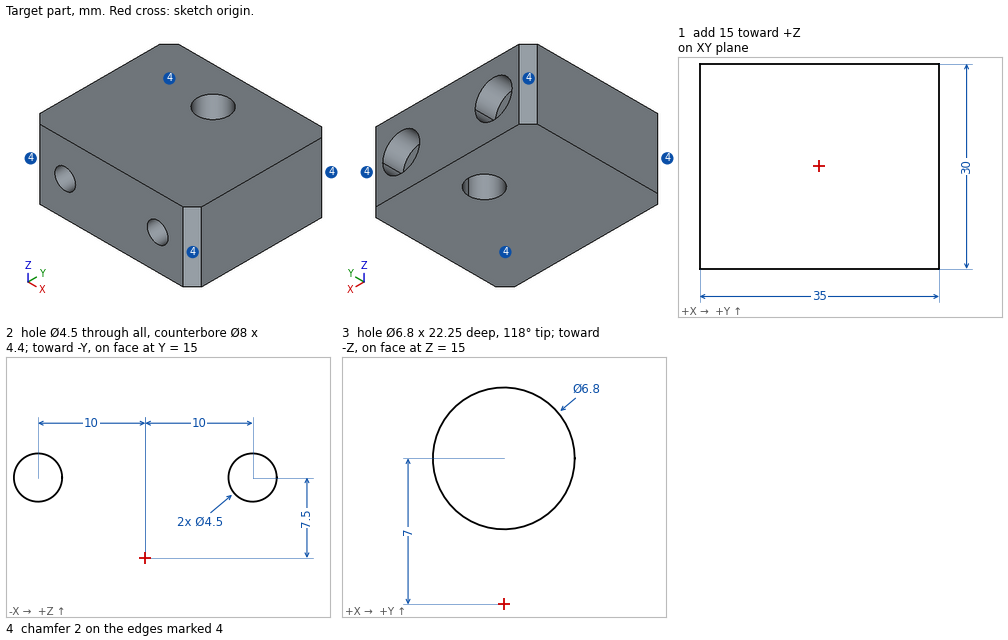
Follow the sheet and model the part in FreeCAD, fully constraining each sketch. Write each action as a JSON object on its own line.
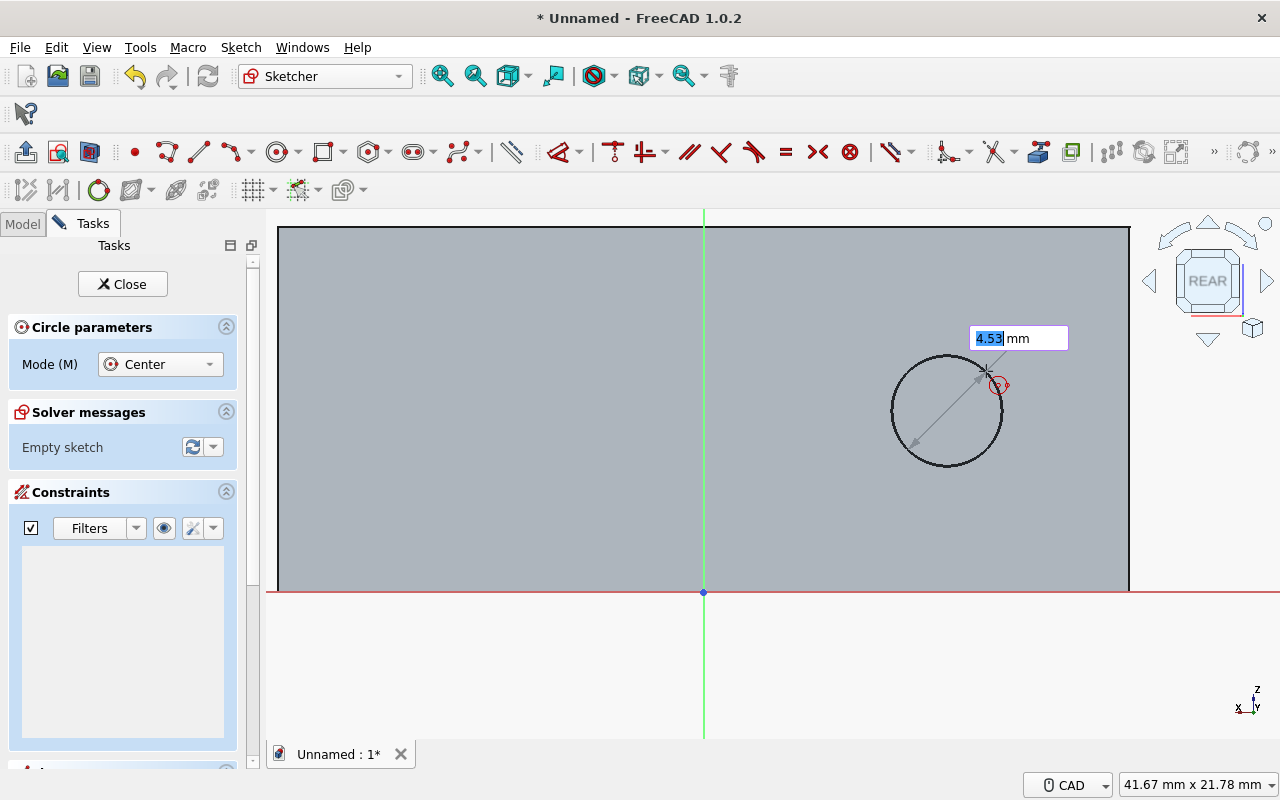
{"action": "type", "text": "4.5"}
{"action": "key", "text": "Return"}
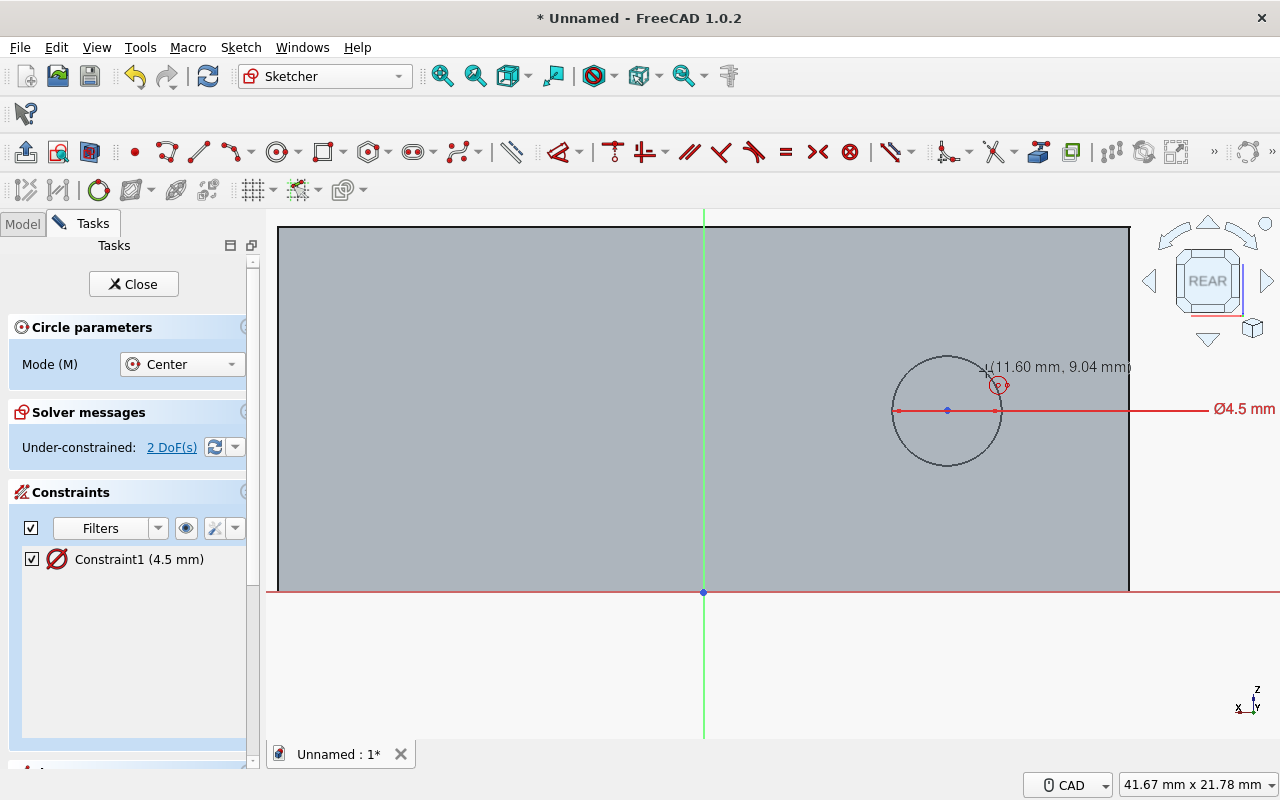
{"action": "left_click", "coordinate": [460, 410]}
{"action": "mouse_move", "coordinate": [499, 371]}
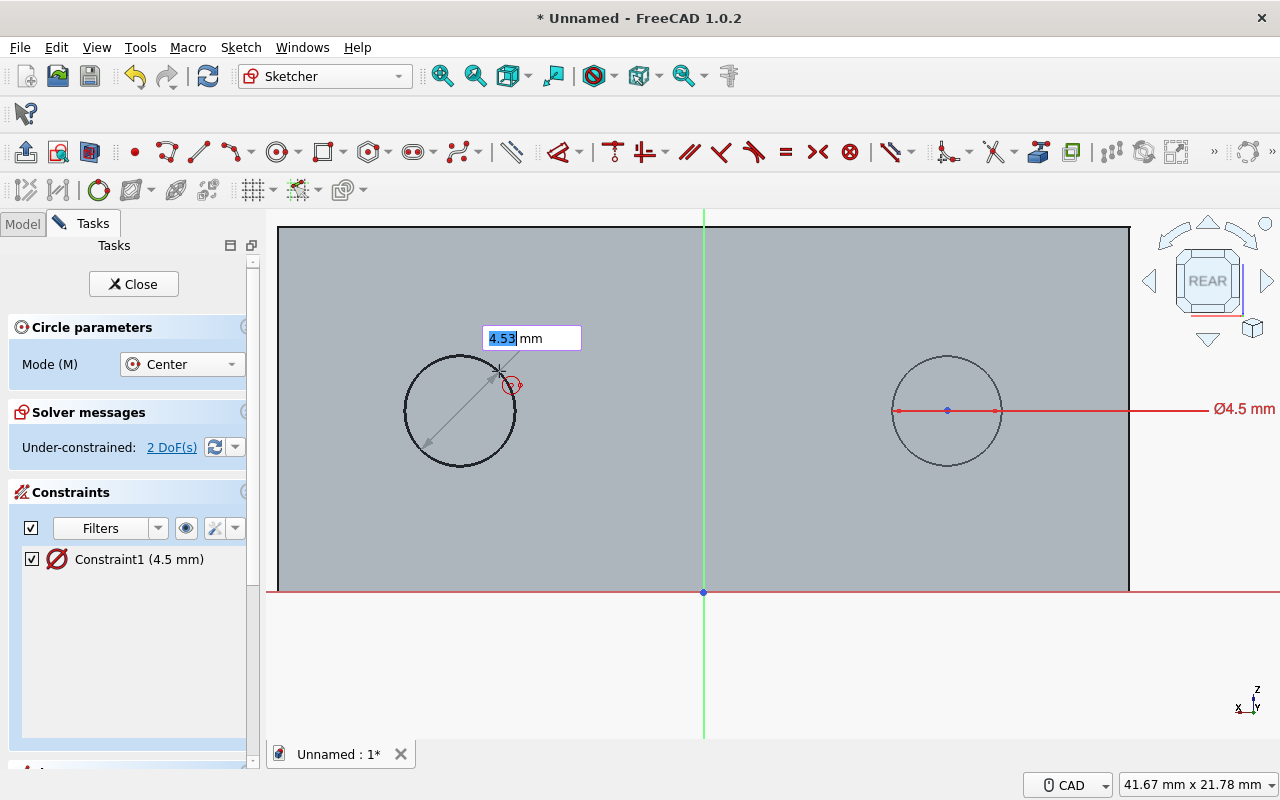
{"action": "type", "text": "4.5"}
{"action": "key", "text": "Return"}
{"action": "key", "text": "Escape"}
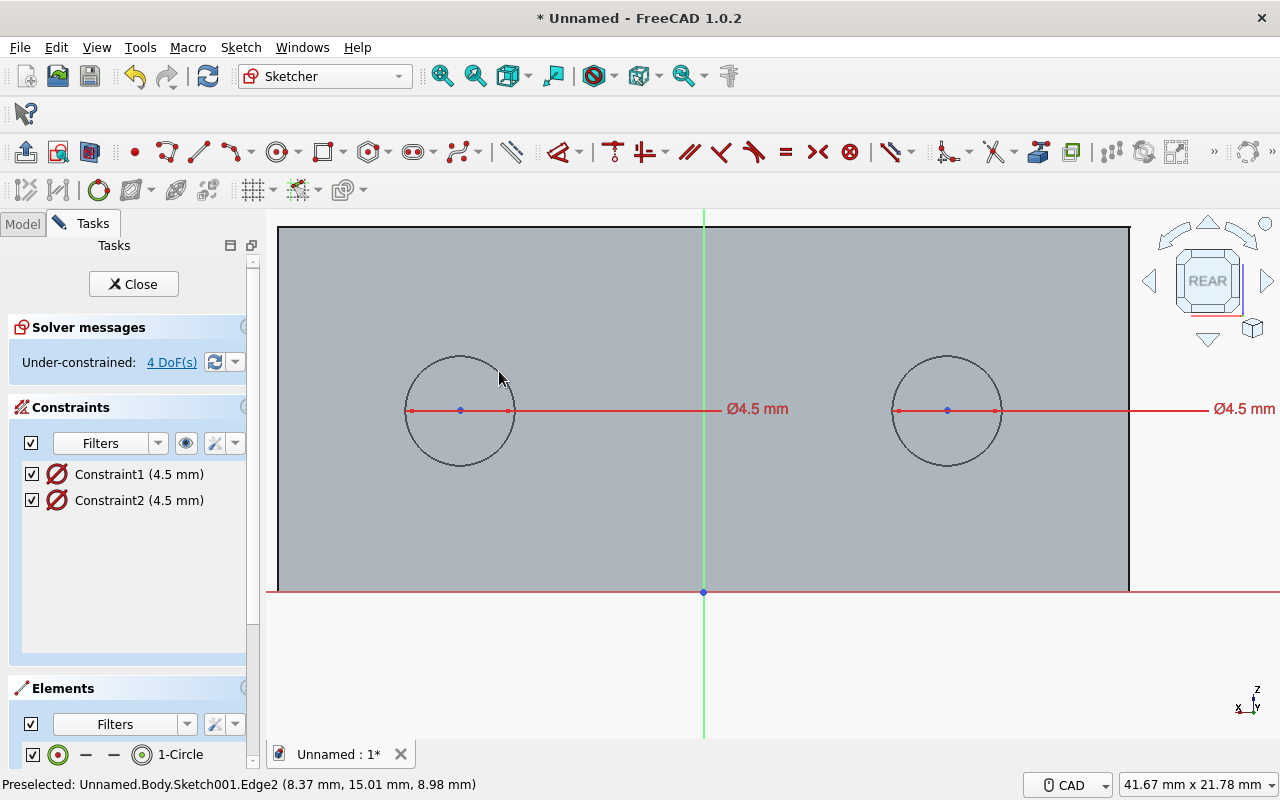
{"action": "left_click", "coordinate": [947, 411]}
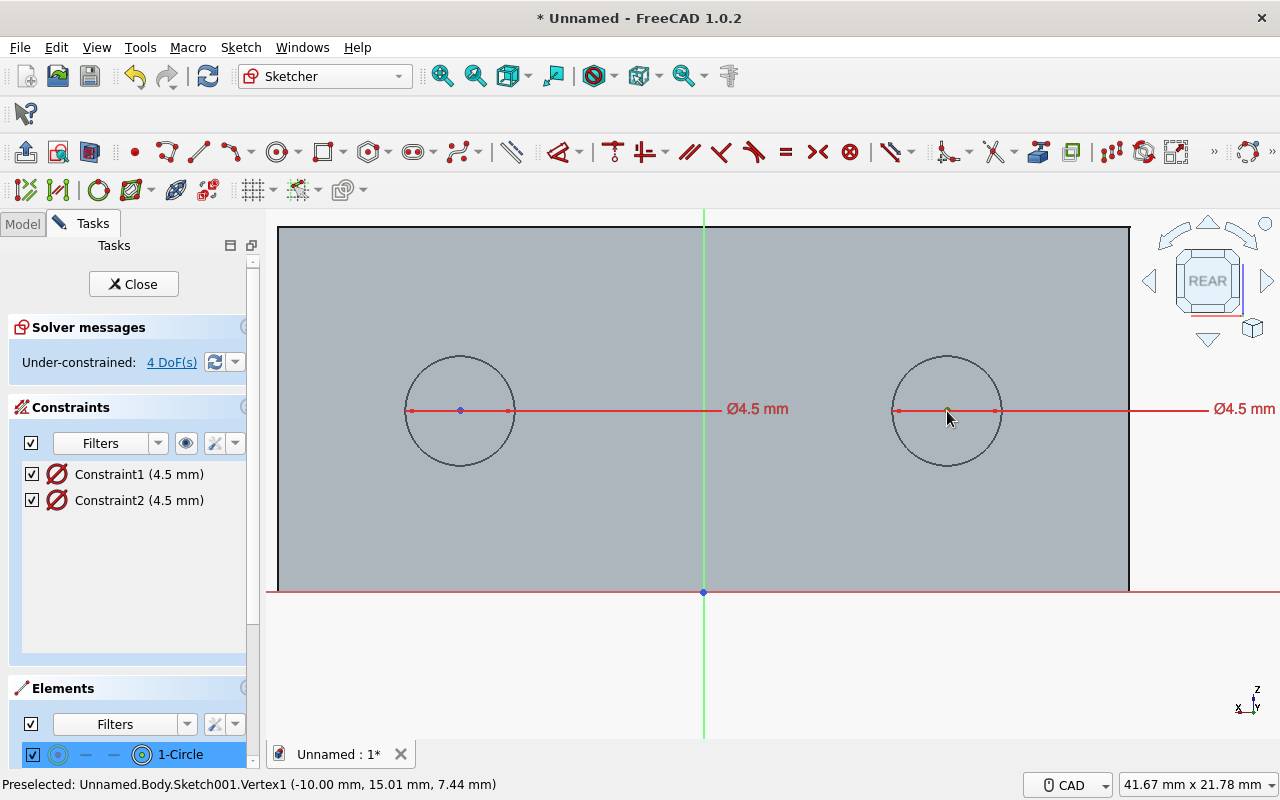
{"action": "left_click", "coordinate": [460, 411]}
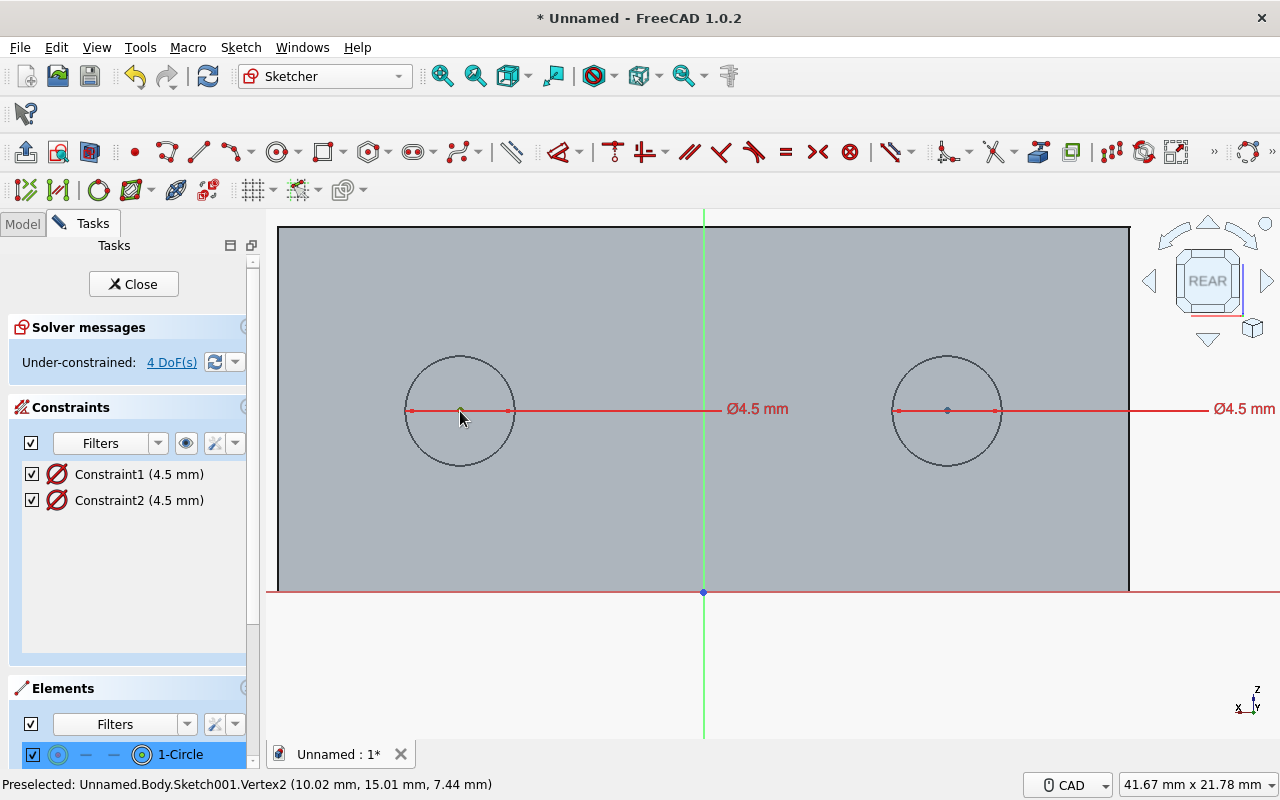
{"action": "left_click", "coordinate": [668, 152]}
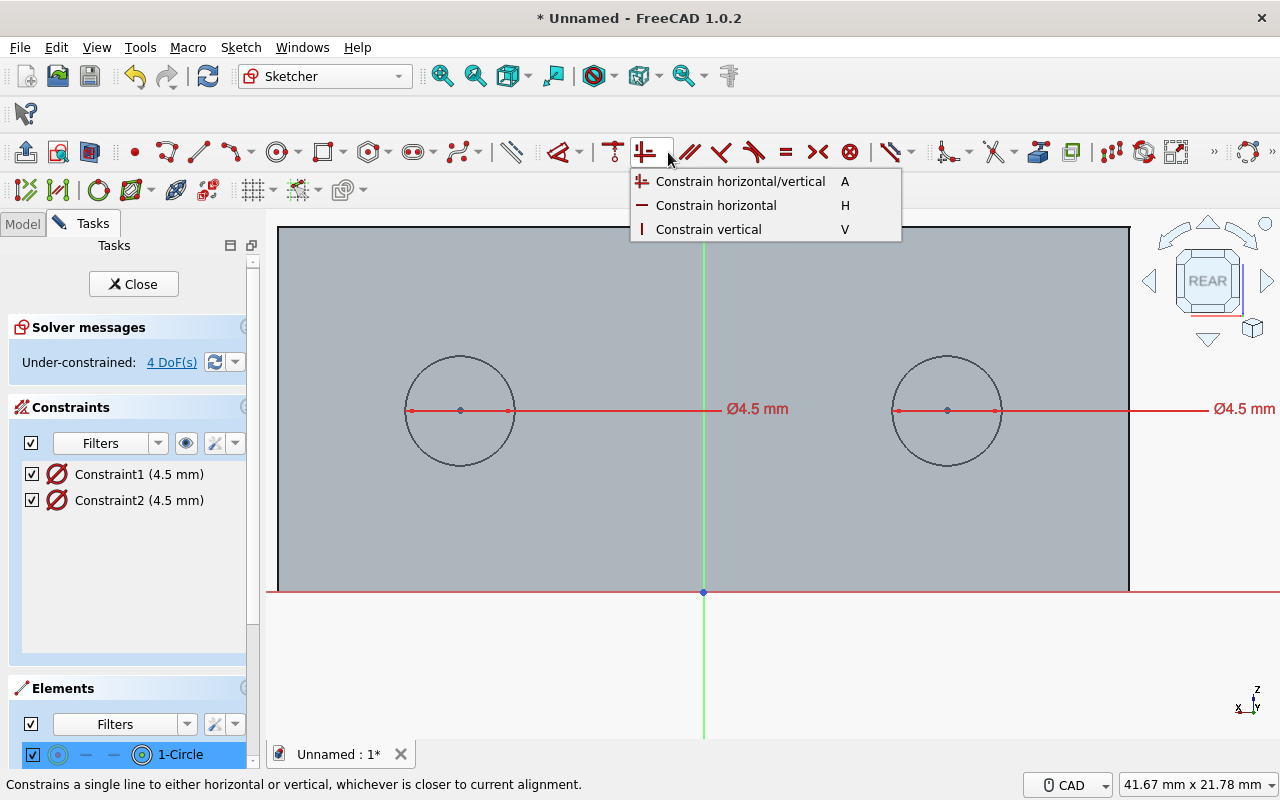
{"action": "left_click", "coordinate": [766, 205]}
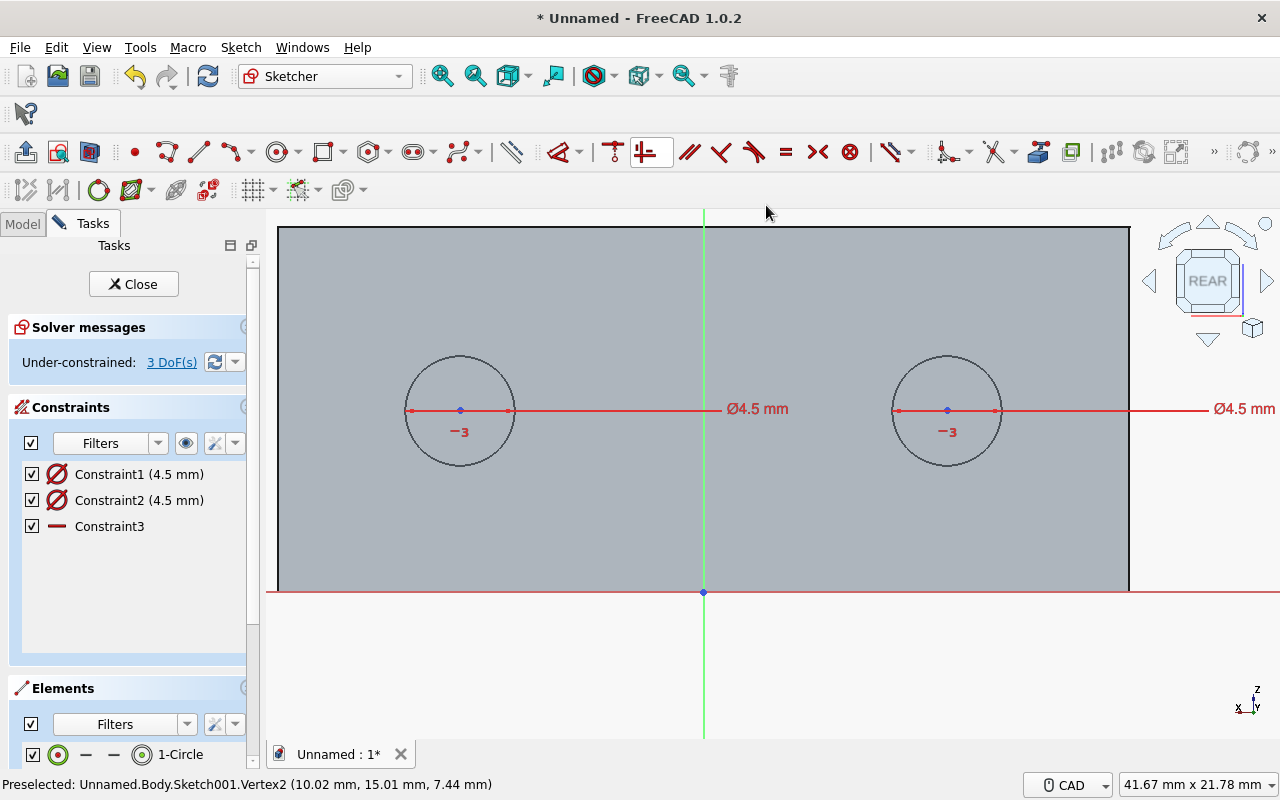
{"action": "key", "text": "d"}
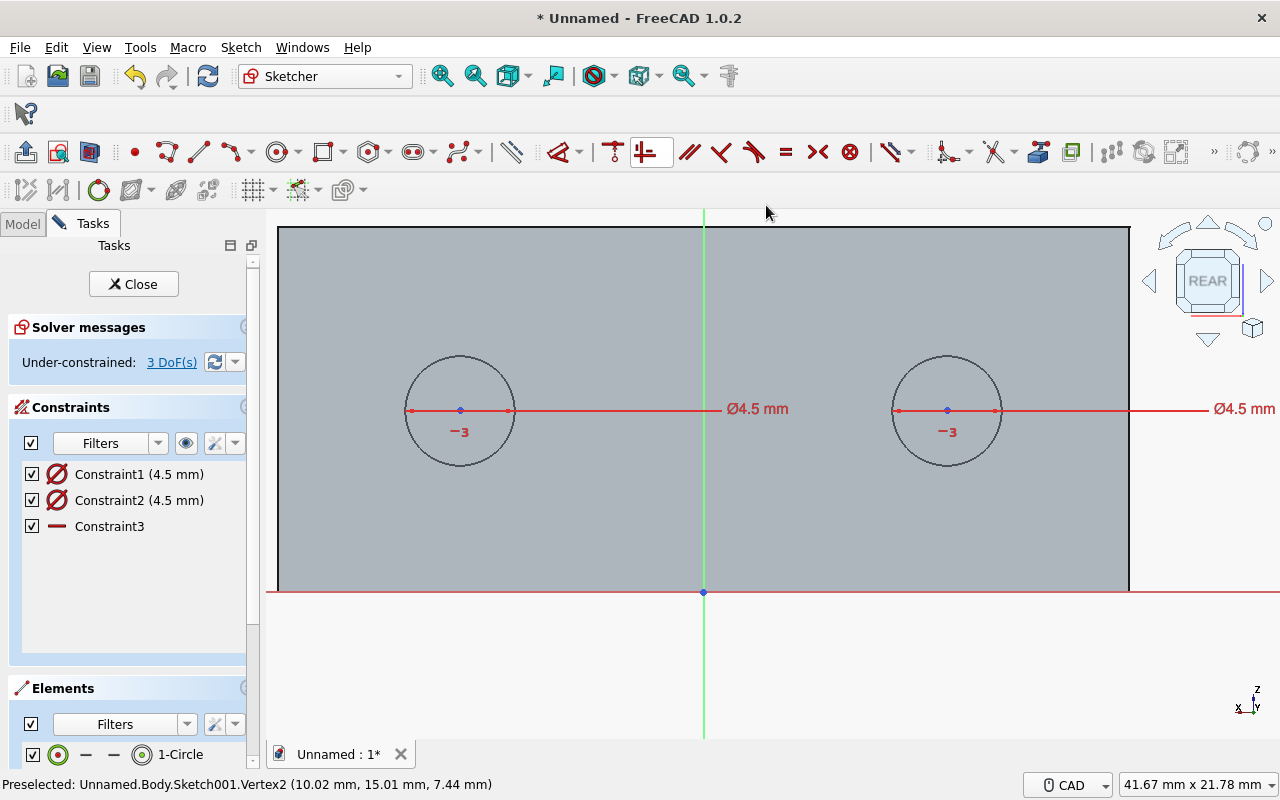
{"action": "left_click", "coordinate": [947, 411]}
{"action": "left_click", "coordinate": [825, 626]}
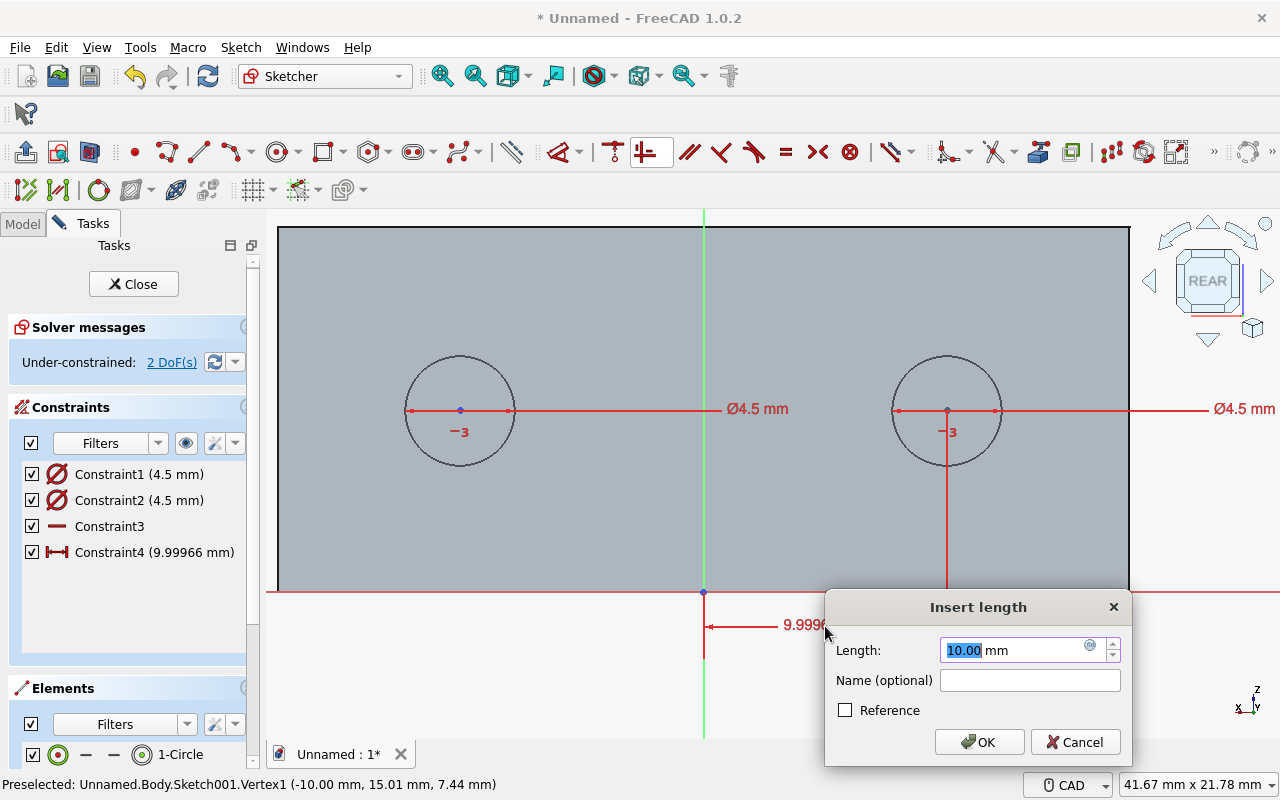
{"action": "type", "text": "10"}
{"action": "key", "text": "Return"}